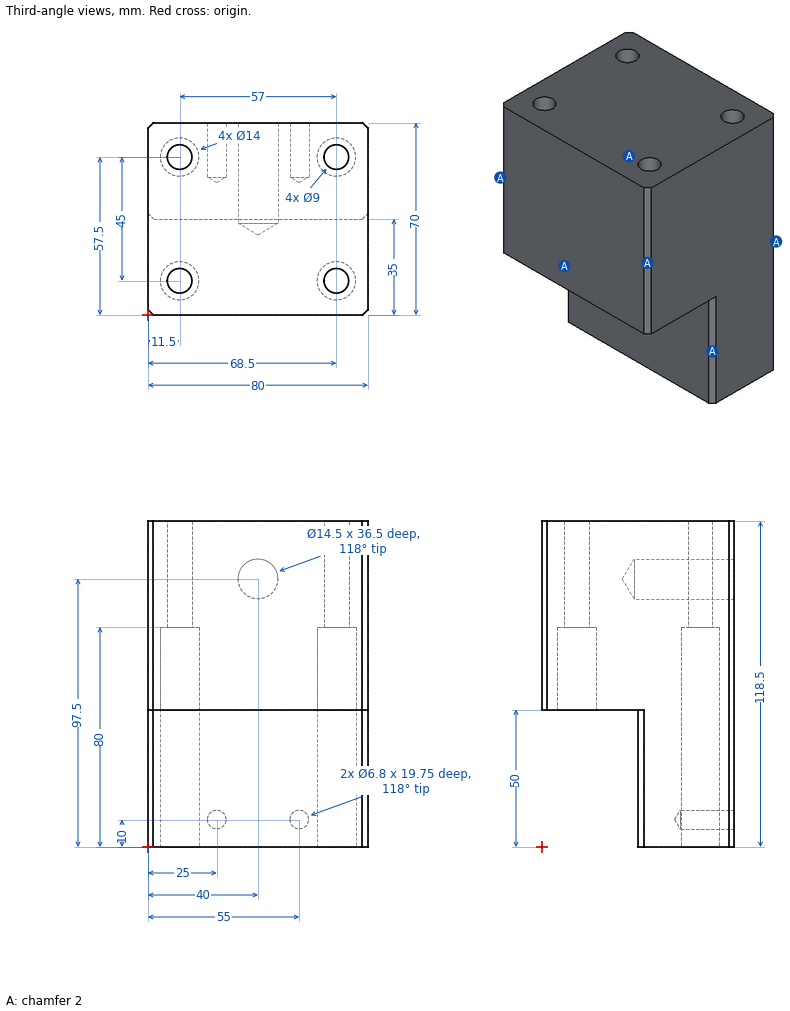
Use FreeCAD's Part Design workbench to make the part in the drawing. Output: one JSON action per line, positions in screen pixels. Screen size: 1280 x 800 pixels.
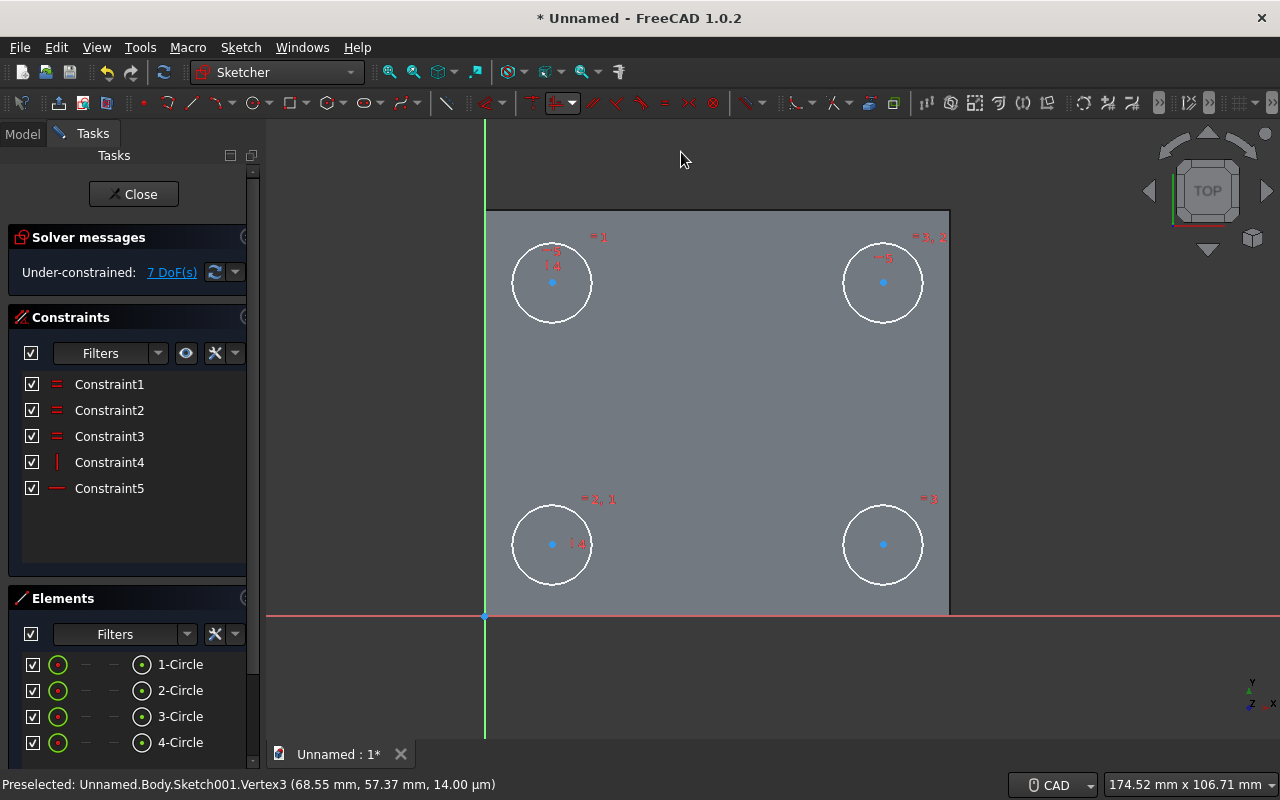
{"action": "left_click", "coordinate": [883, 283]}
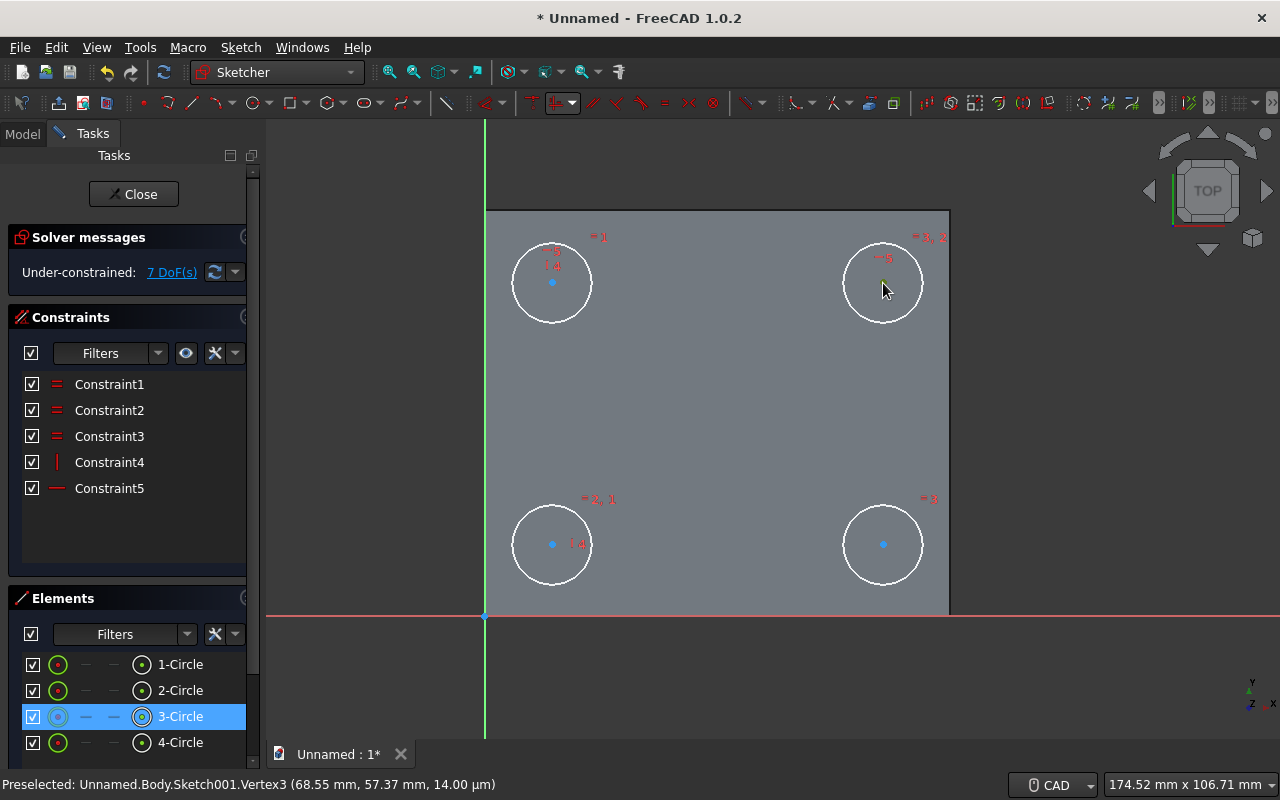
{"action": "left_click", "coordinate": [883, 545]}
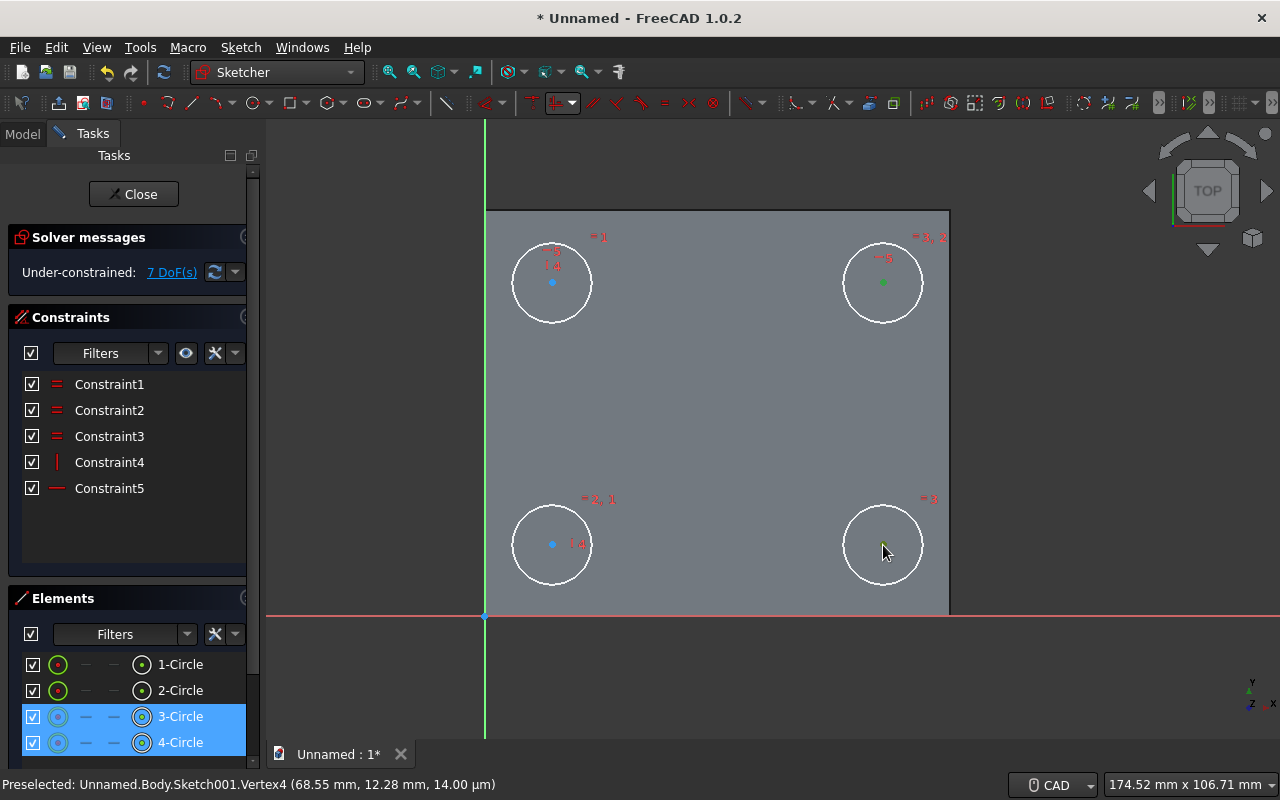
{"action": "key", "text": "v"}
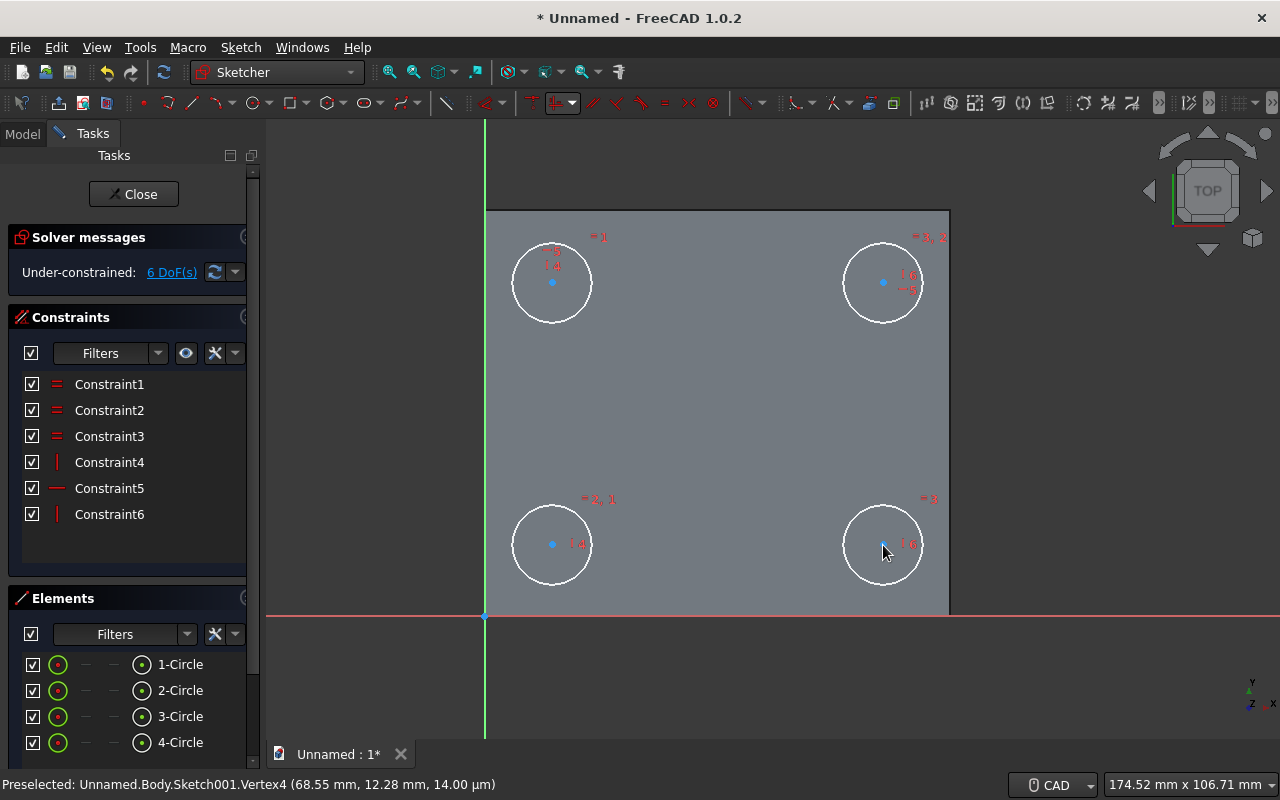
{"action": "left_click", "coordinate": [552, 545]}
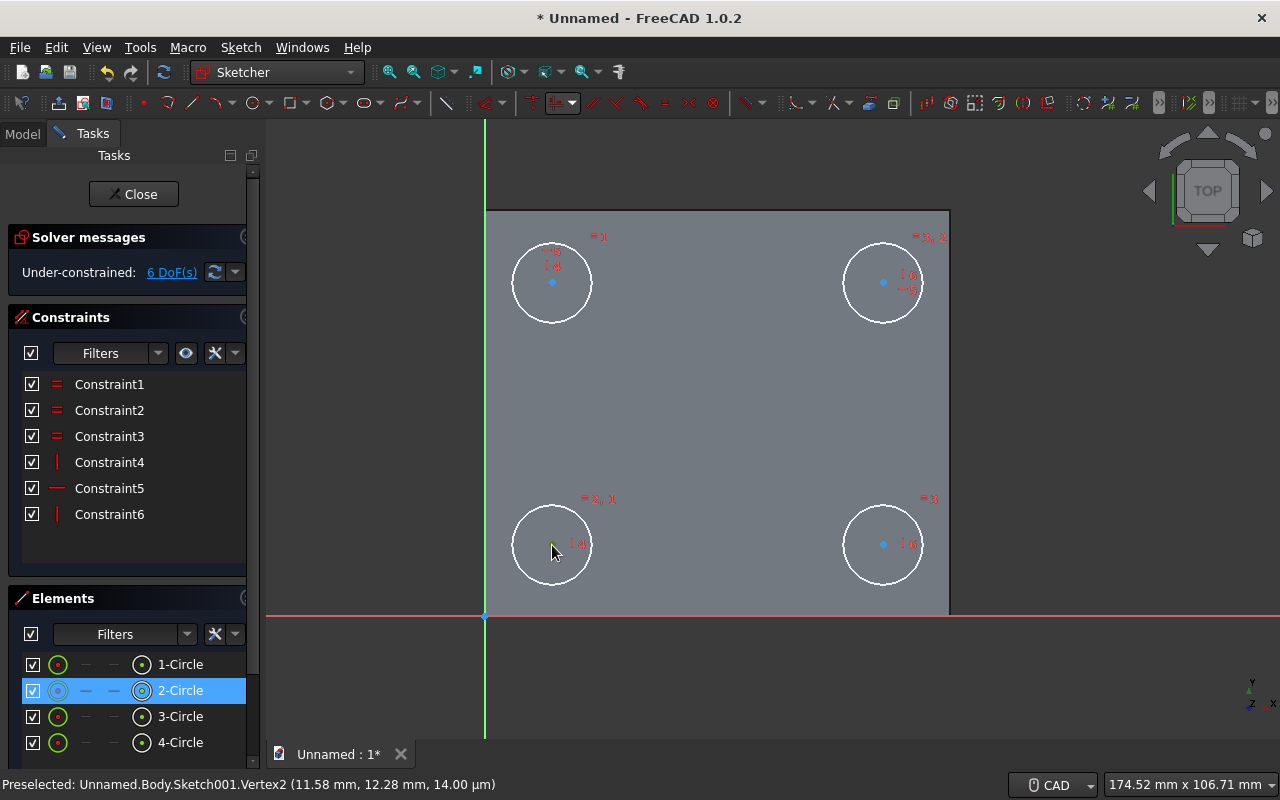
{"action": "left_click", "coordinate": [883, 545]}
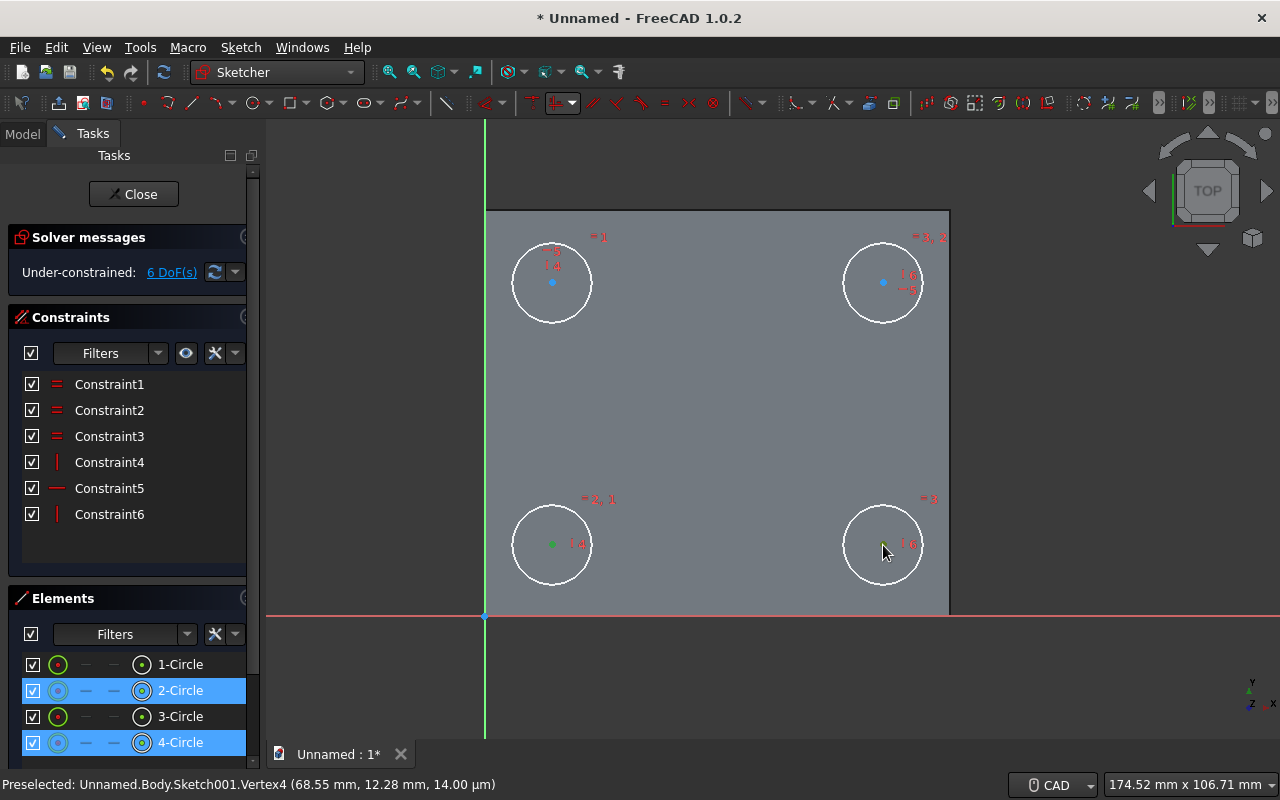
{"action": "left_click", "coordinate": [574, 104]}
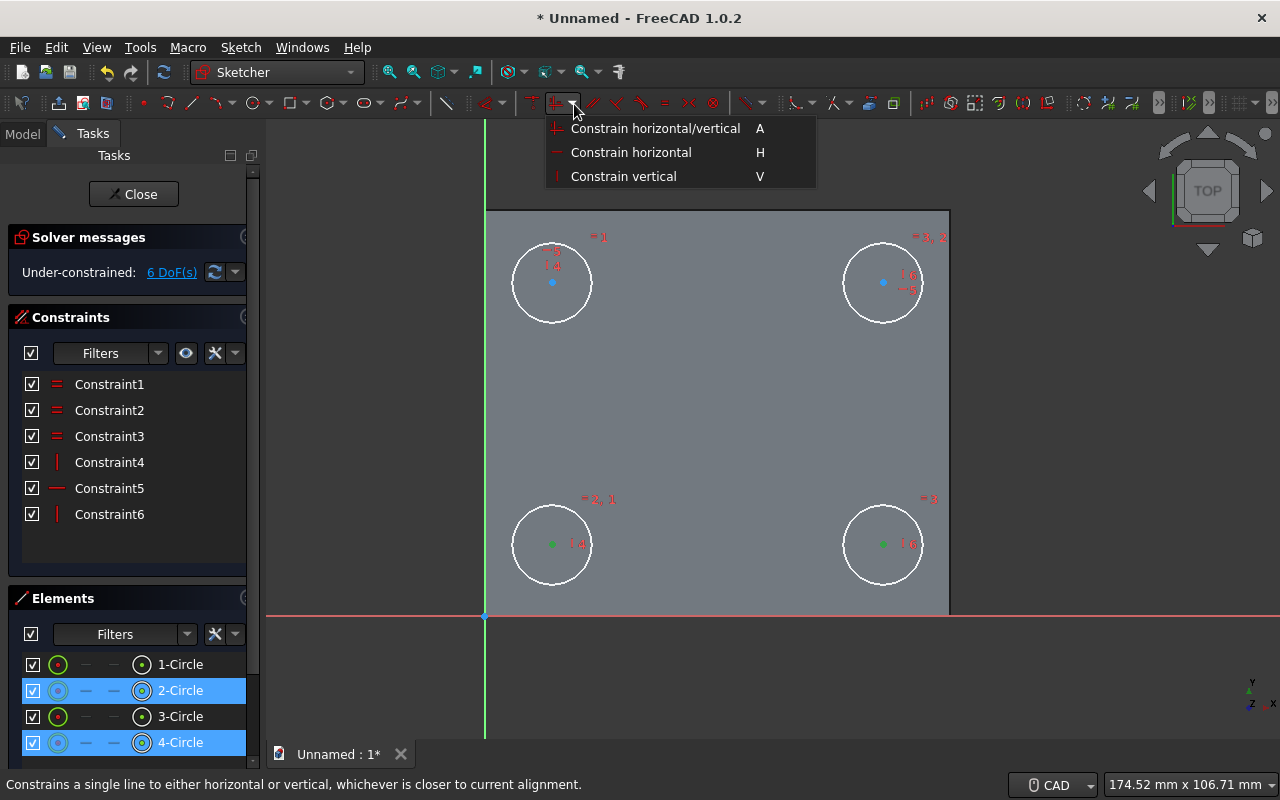
{"action": "left_click", "coordinate": [681, 152]}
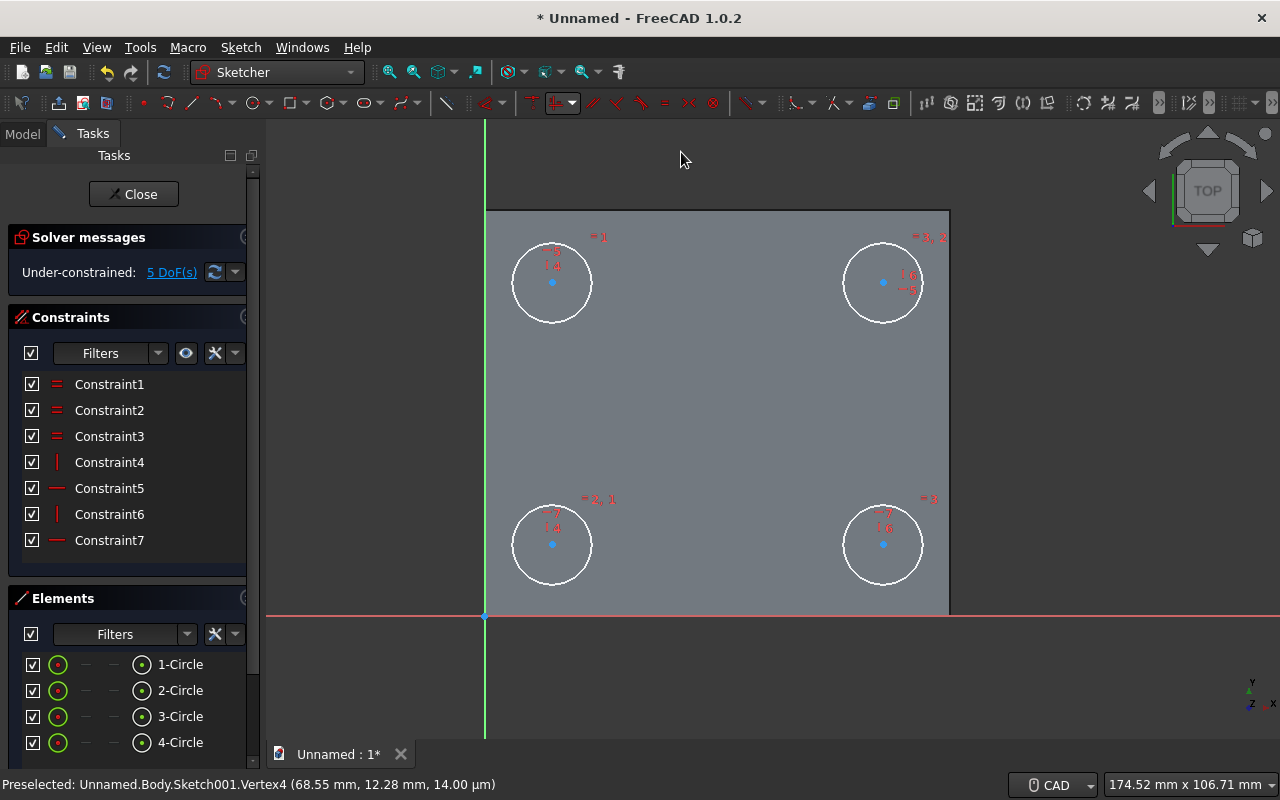
{"action": "key", "text": "d"}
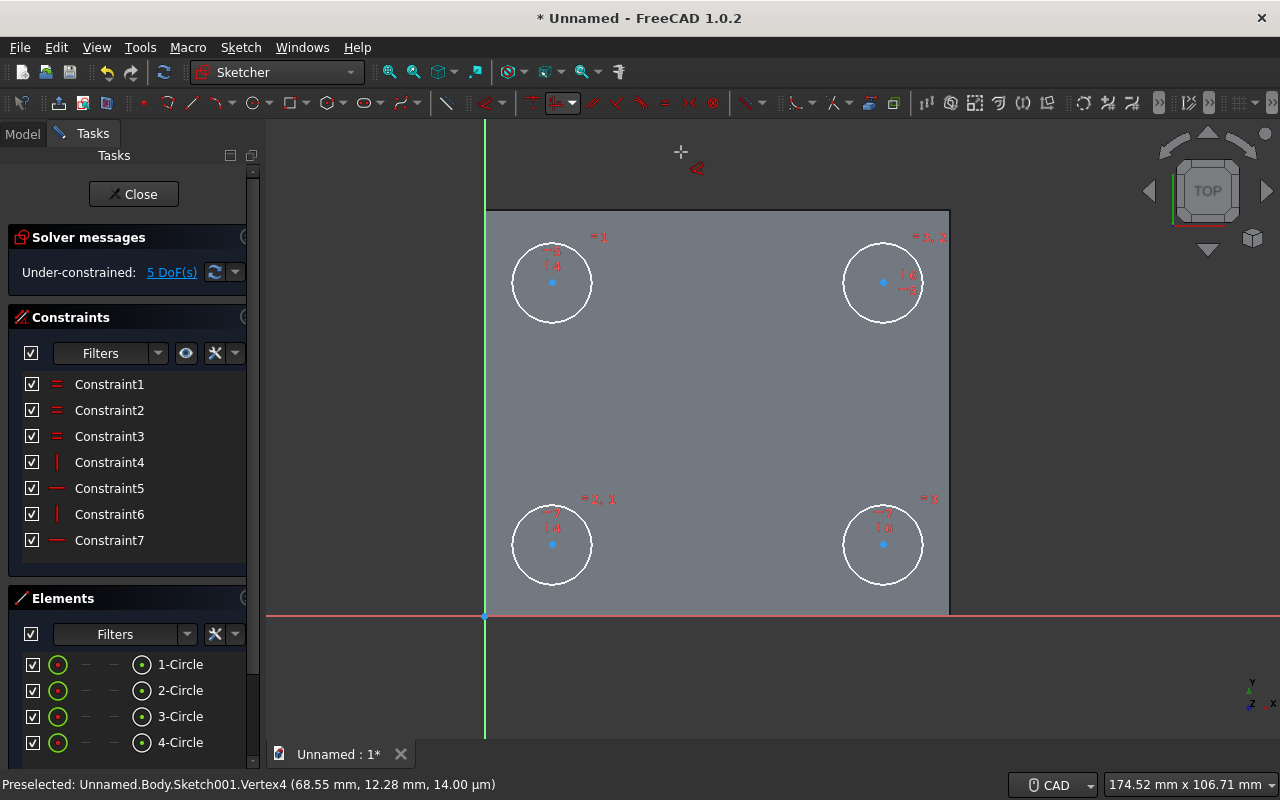
{"action": "left_click", "coordinate": [580, 255]}
{"action": "left_click", "coordinate": [603, 232]}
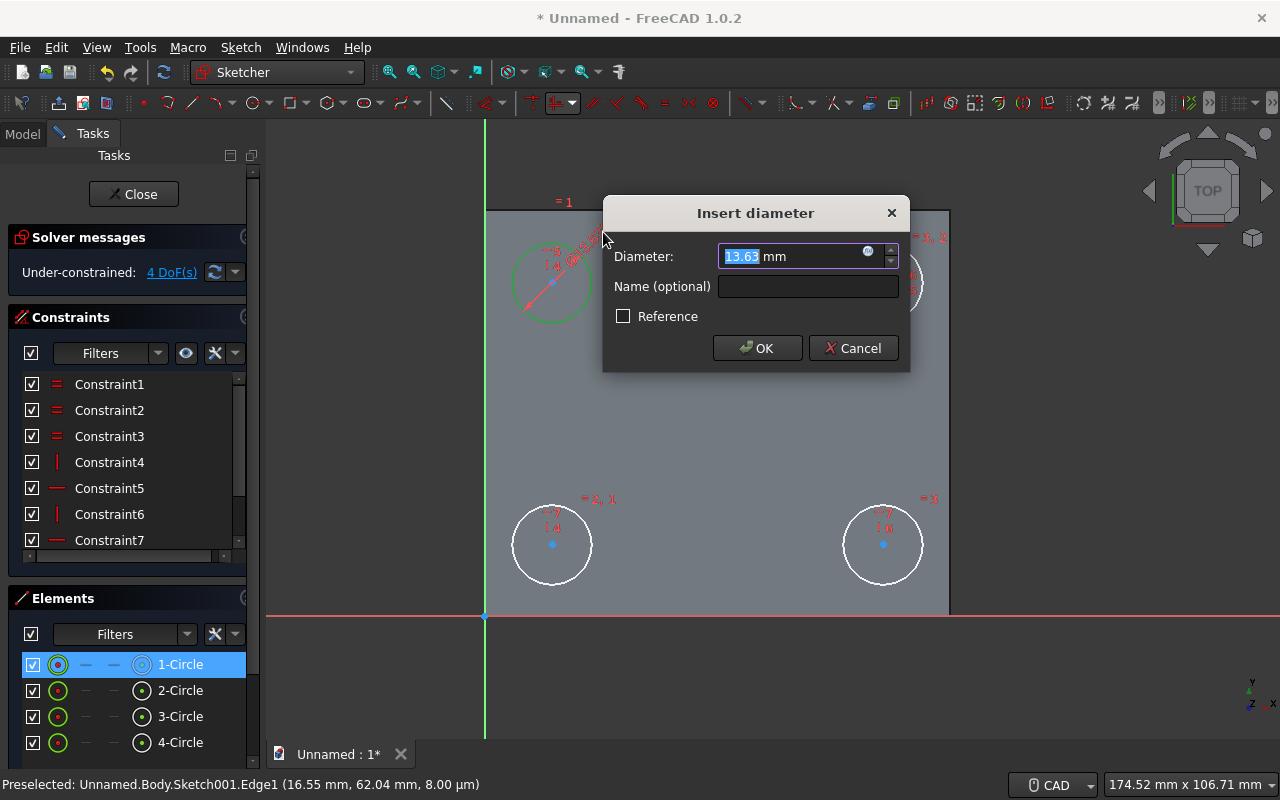
{"action": "type", "text": "14"}
{"action": "key", "text": "Return"}